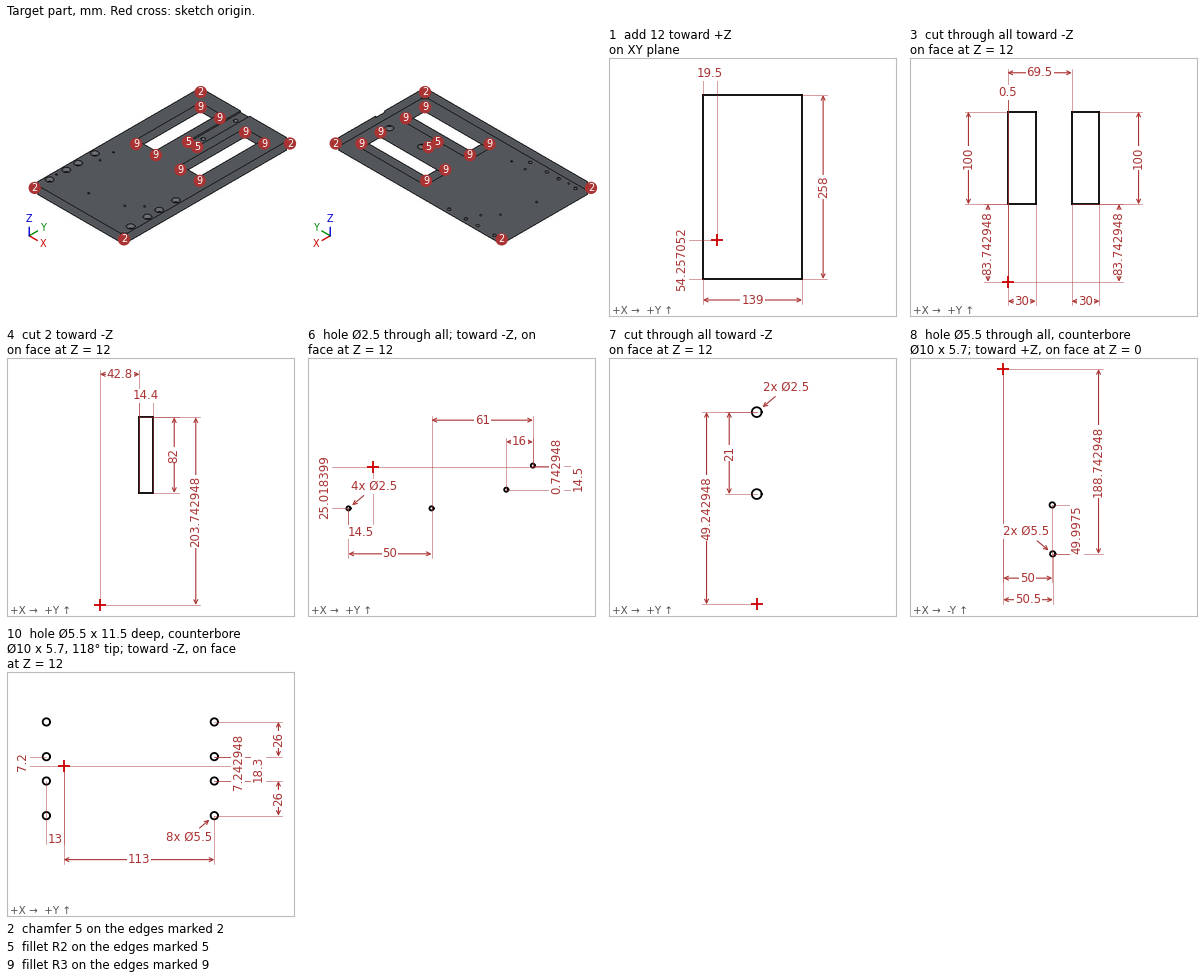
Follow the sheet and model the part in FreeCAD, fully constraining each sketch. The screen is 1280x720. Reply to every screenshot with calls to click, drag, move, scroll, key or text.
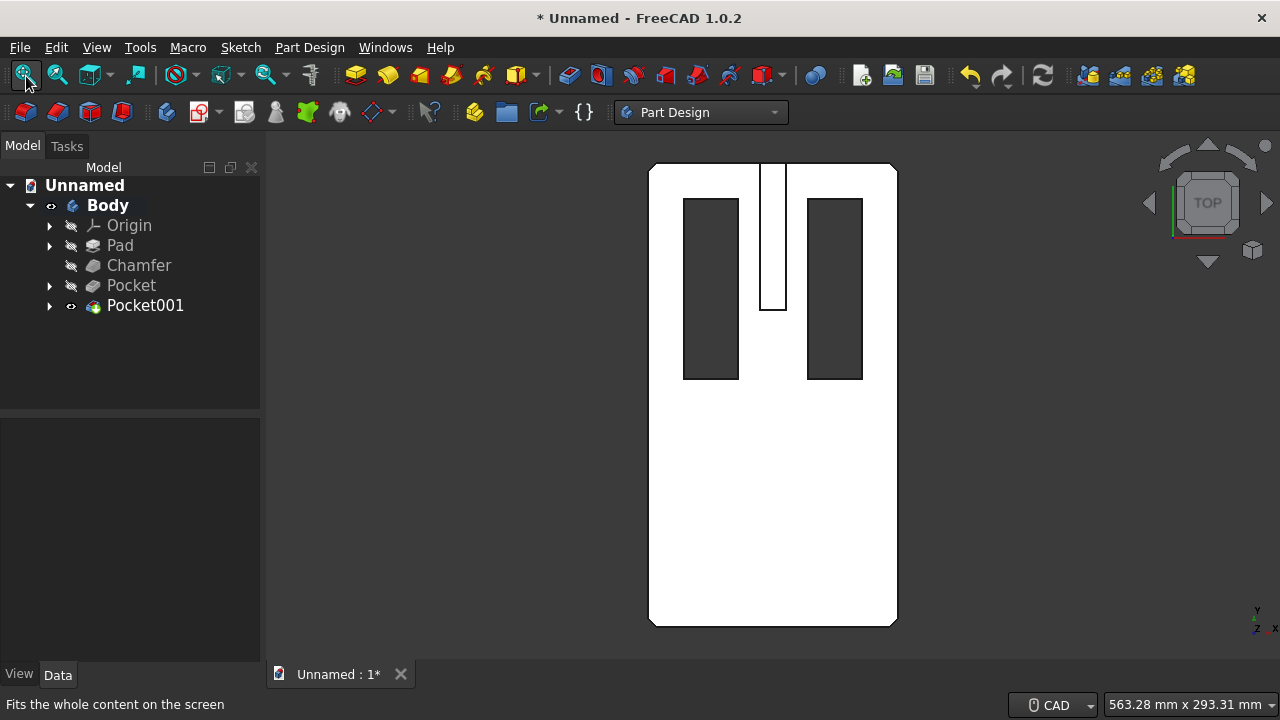
key(0)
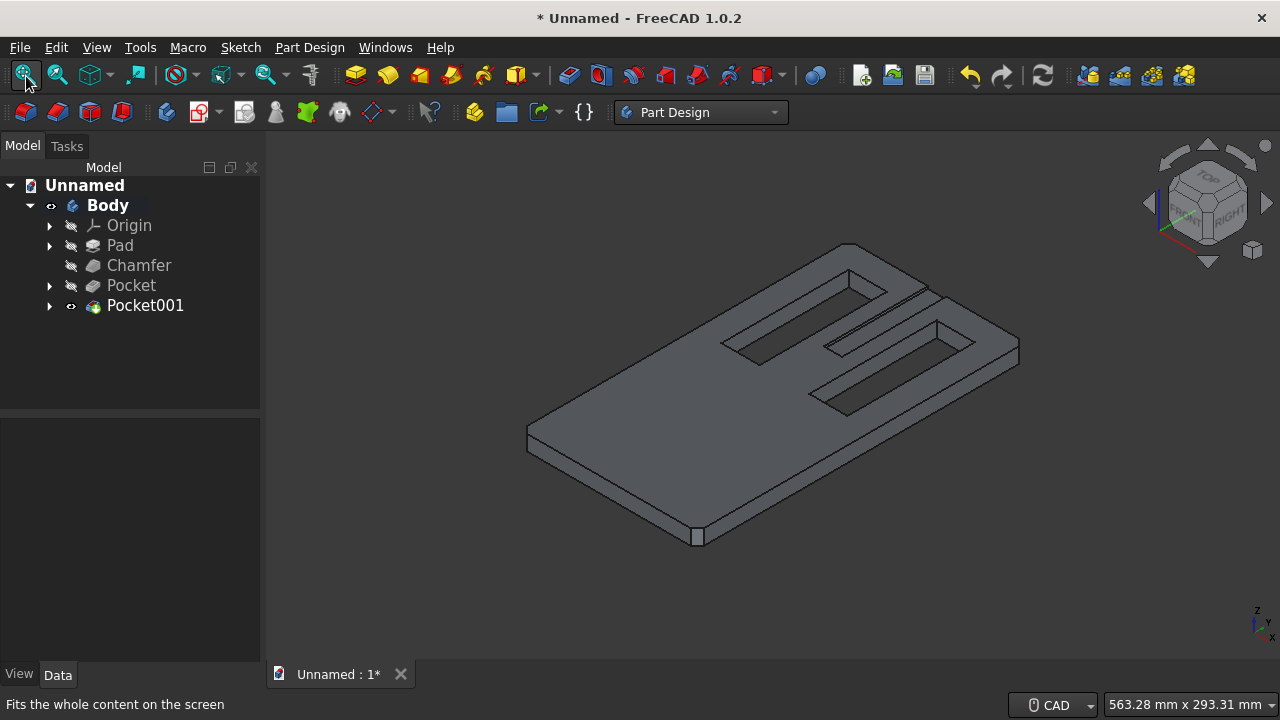
scroll(842, 357, up, 13)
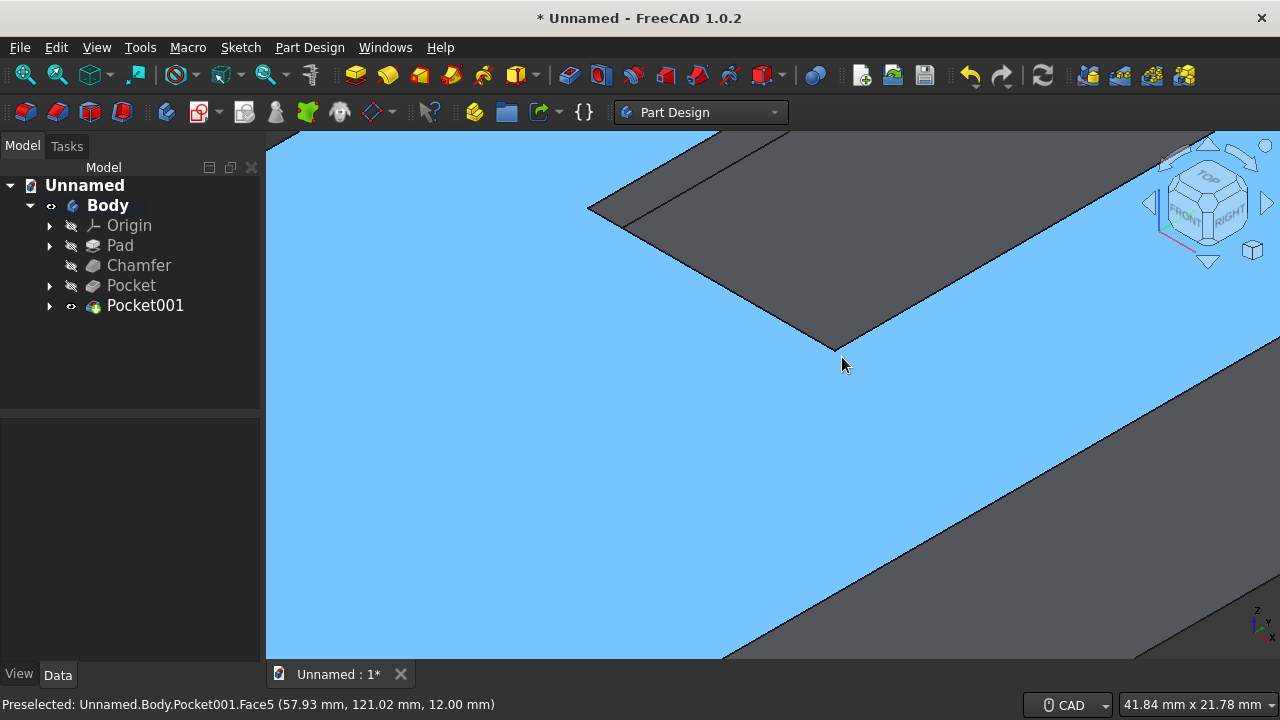
key(v)
key(f)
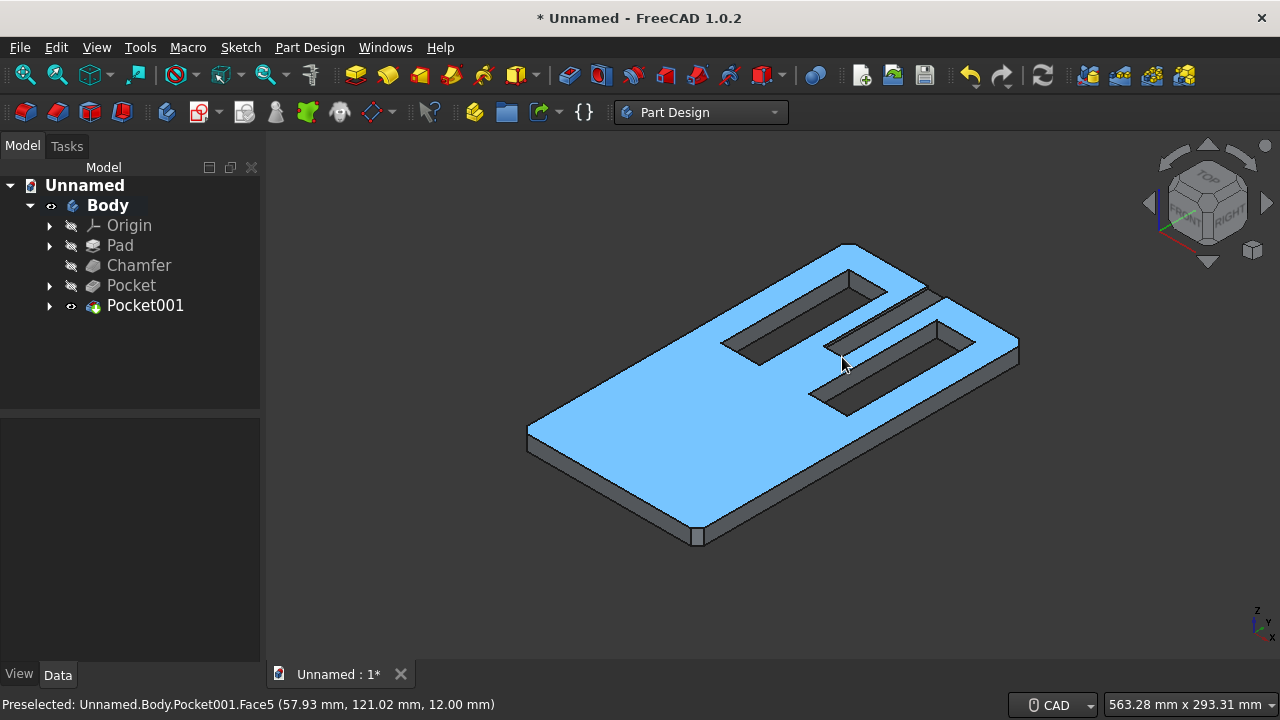
key(1)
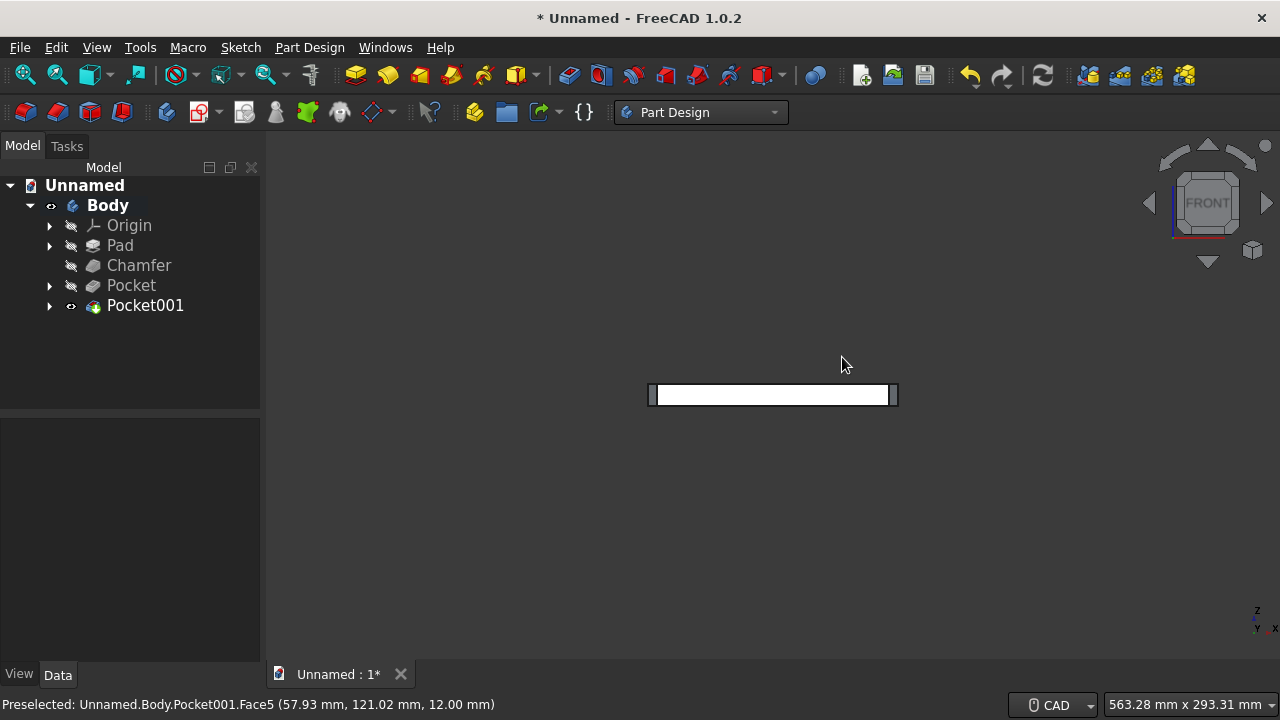
click(26, 76)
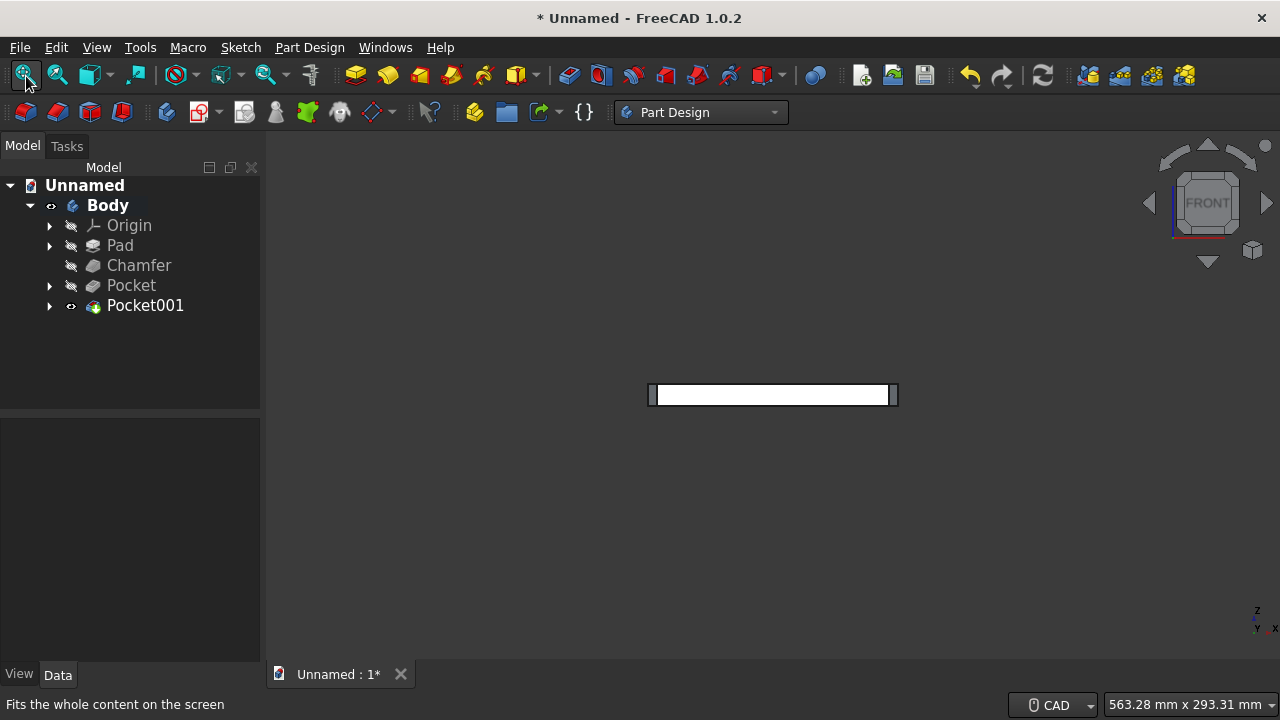
scroll(786, 385, up, 13)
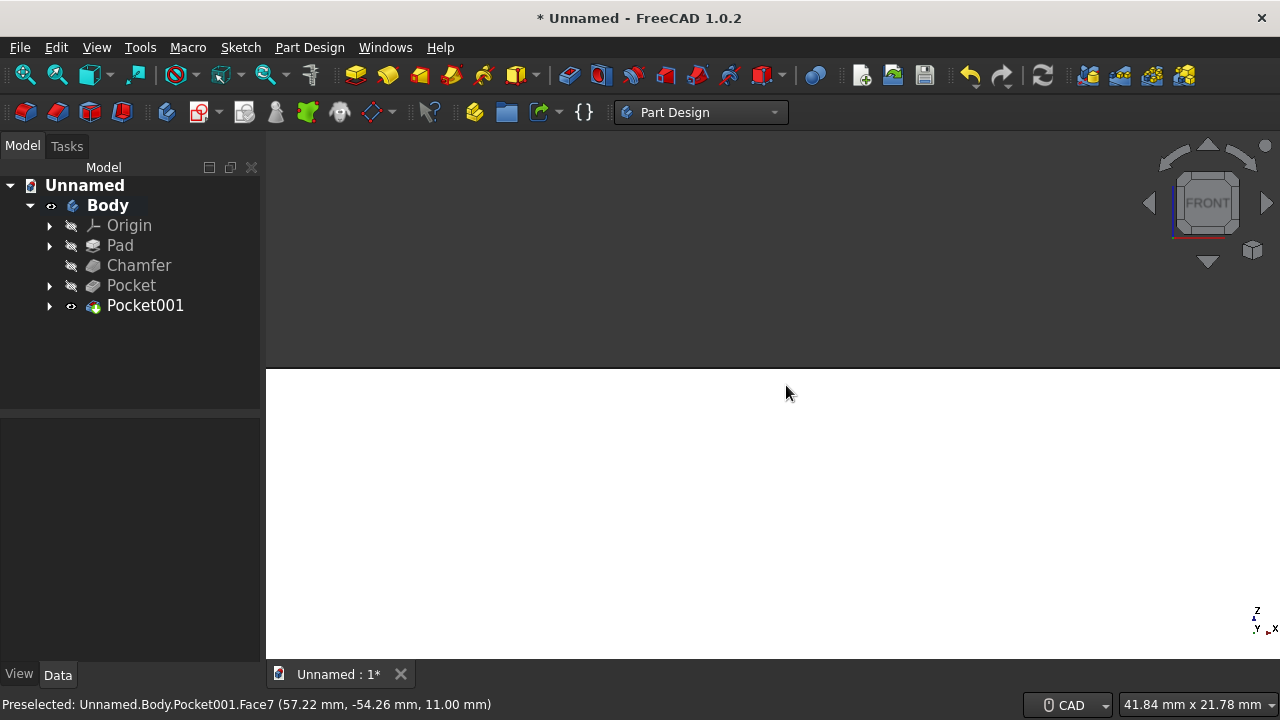
key(v)
key(f)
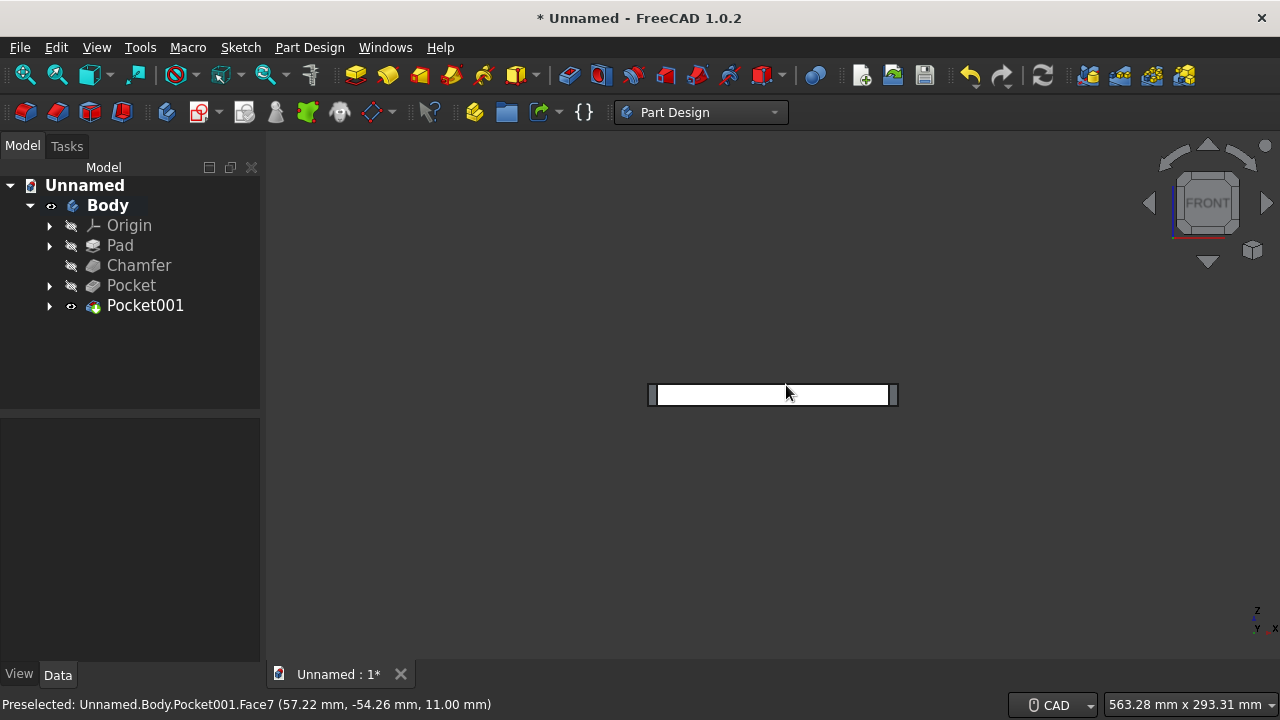
key(3)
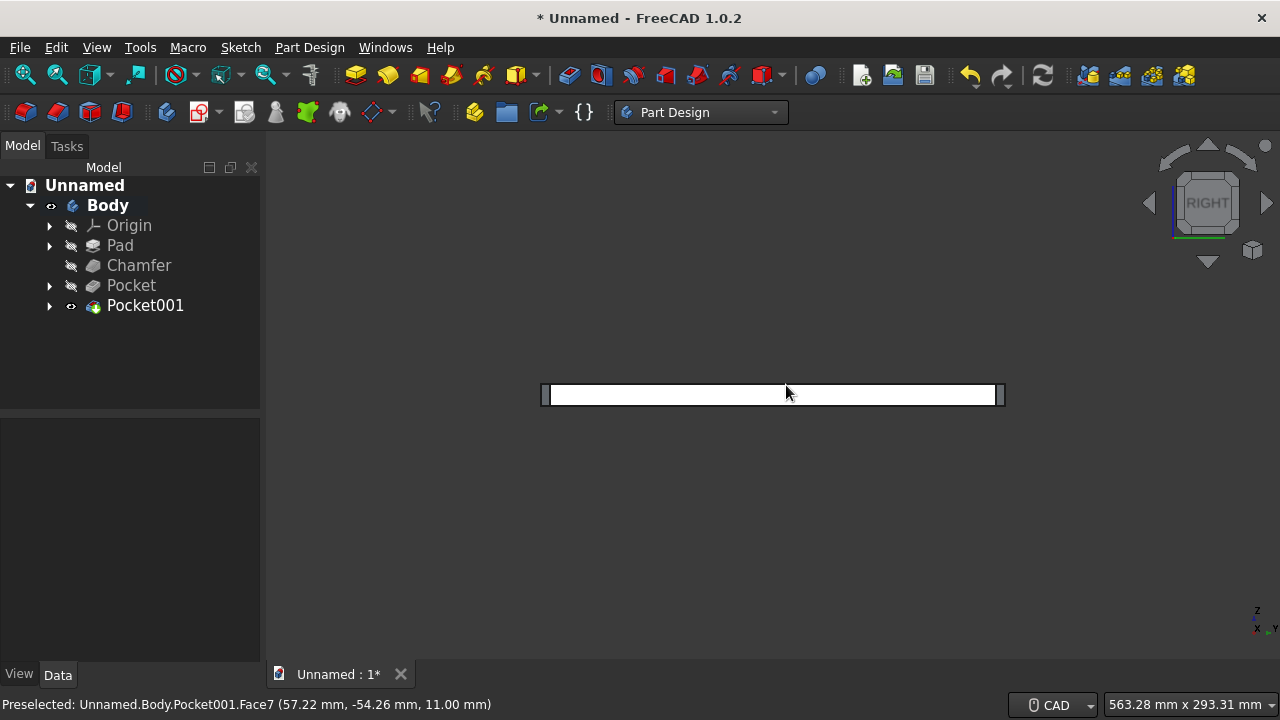
scroll(858, 385, up, 13)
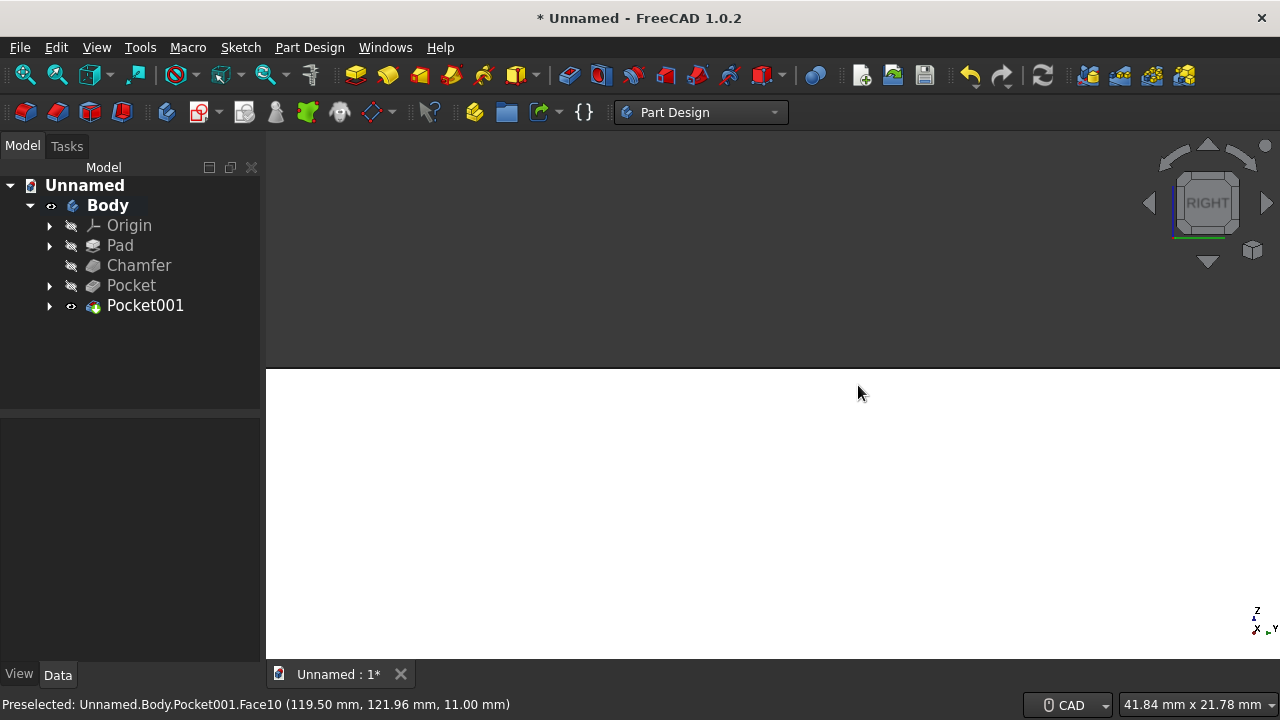
key(v)
key(f)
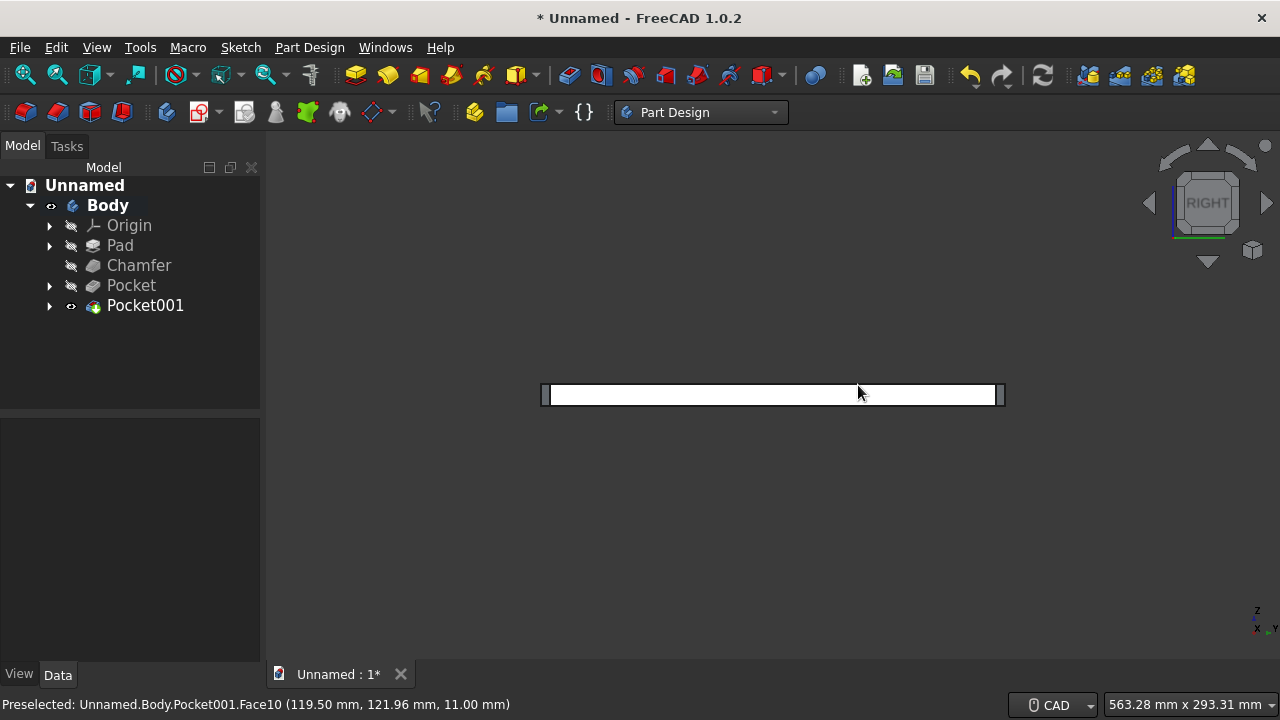
key(5)